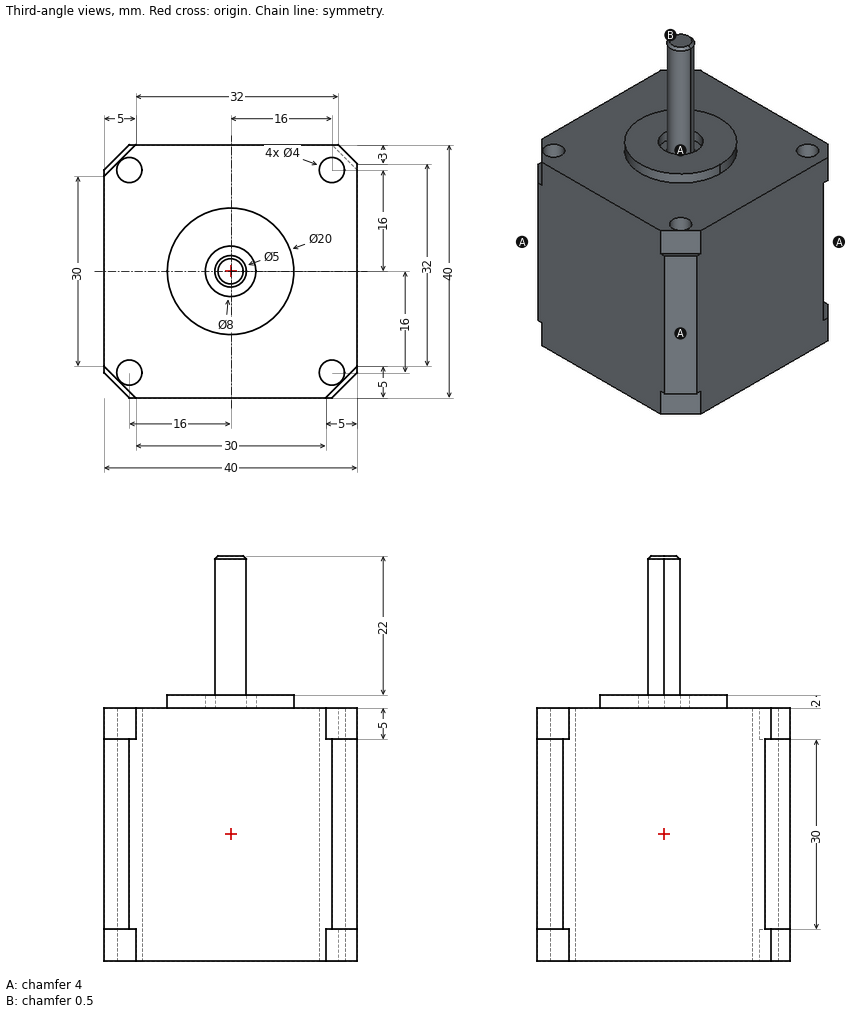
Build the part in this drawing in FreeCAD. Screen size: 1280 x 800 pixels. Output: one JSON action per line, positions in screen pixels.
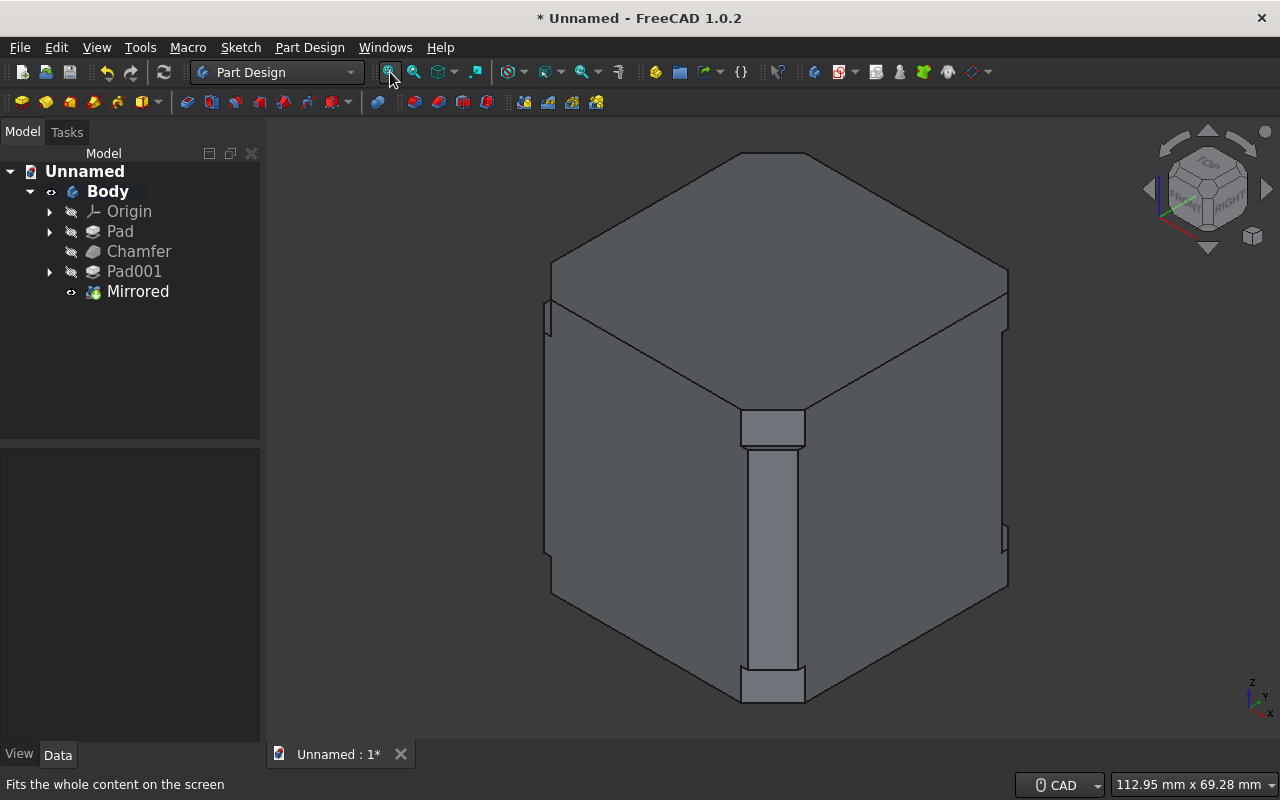
{"action": "left_click", "coordinate": [773, 280]}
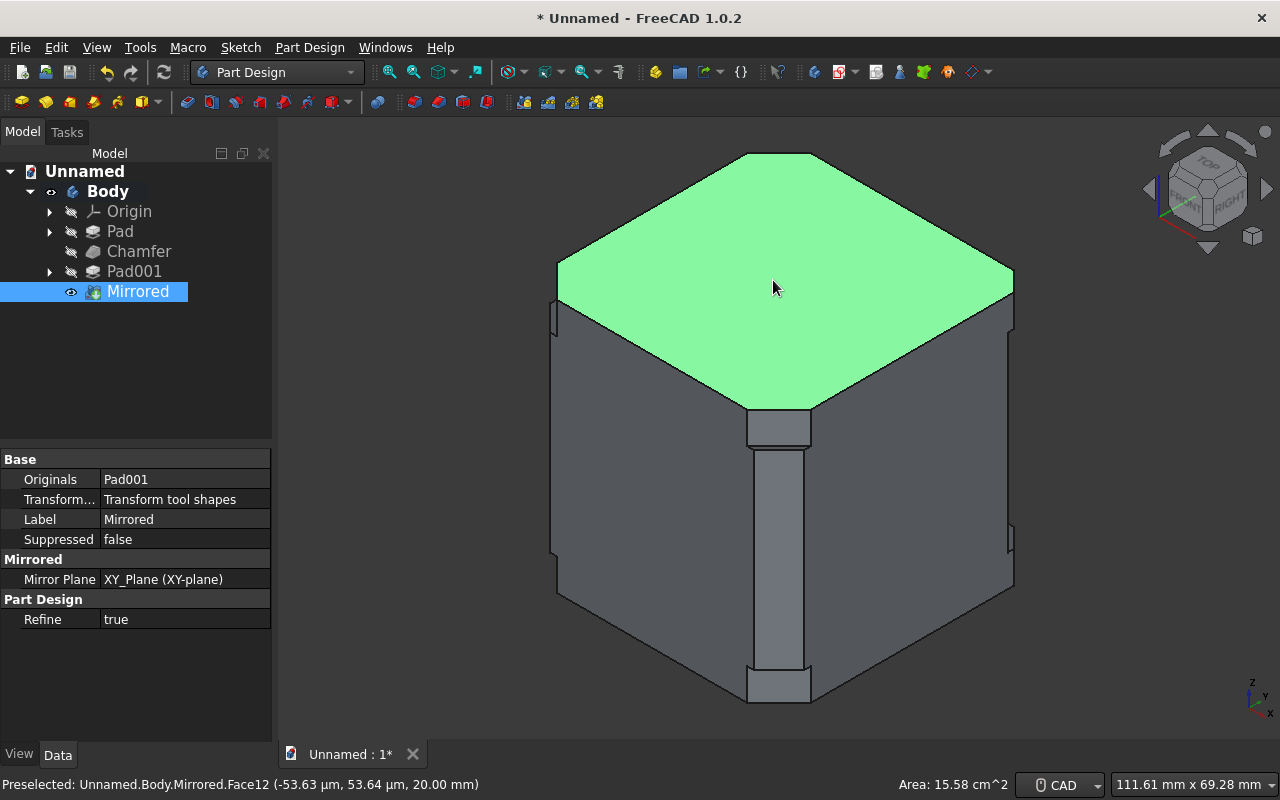
{"action": "left_click", "coordinate": [840, 72]}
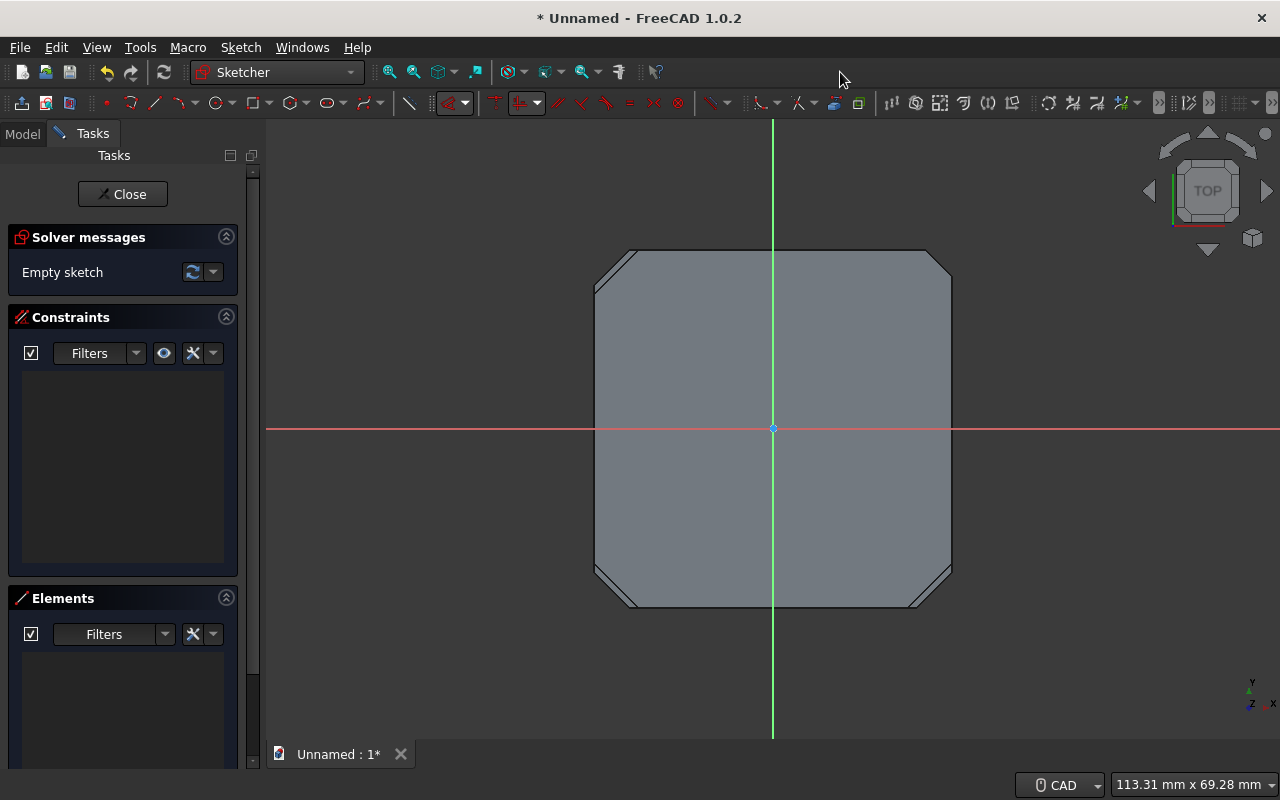
{"action": "scroll", "coordinate": [829, 429], "scroll_direction": "up", "scroll_amount": 4}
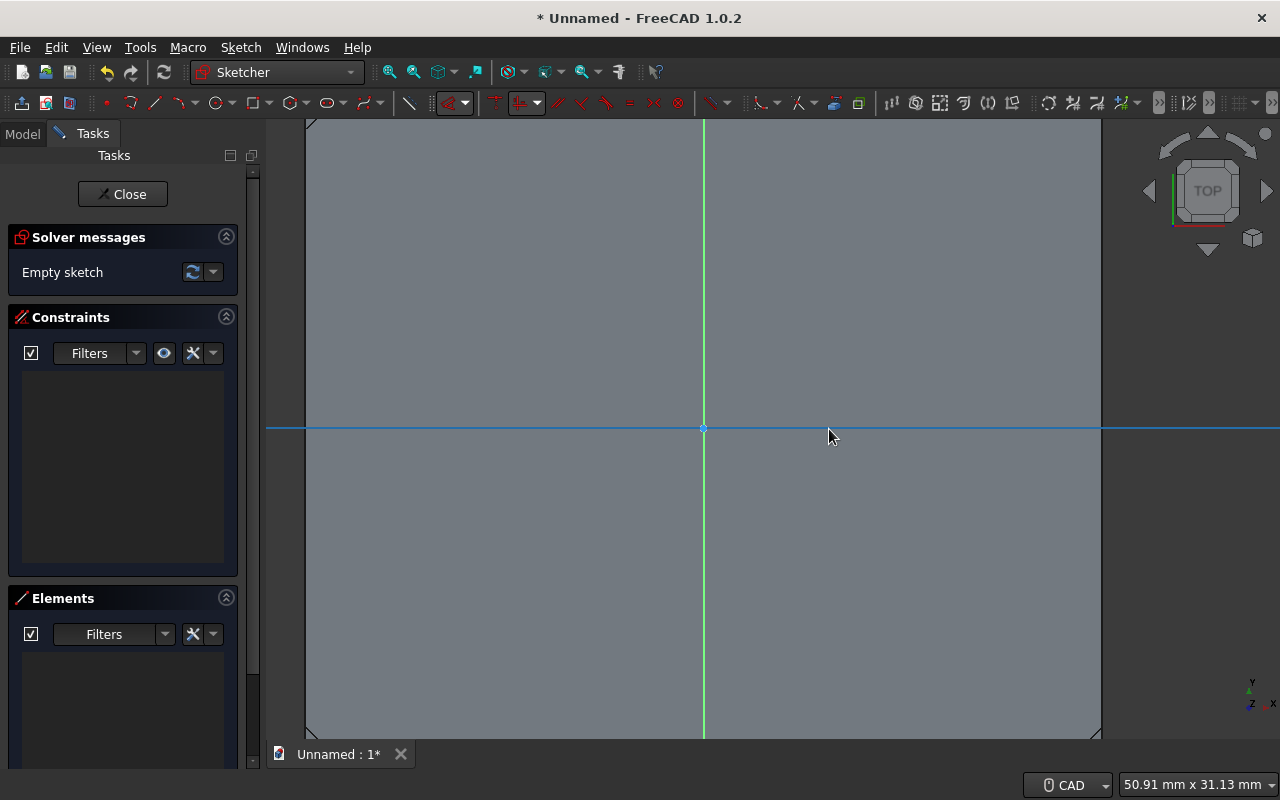
{"action": "left_click", "coordinate": [216, 104]}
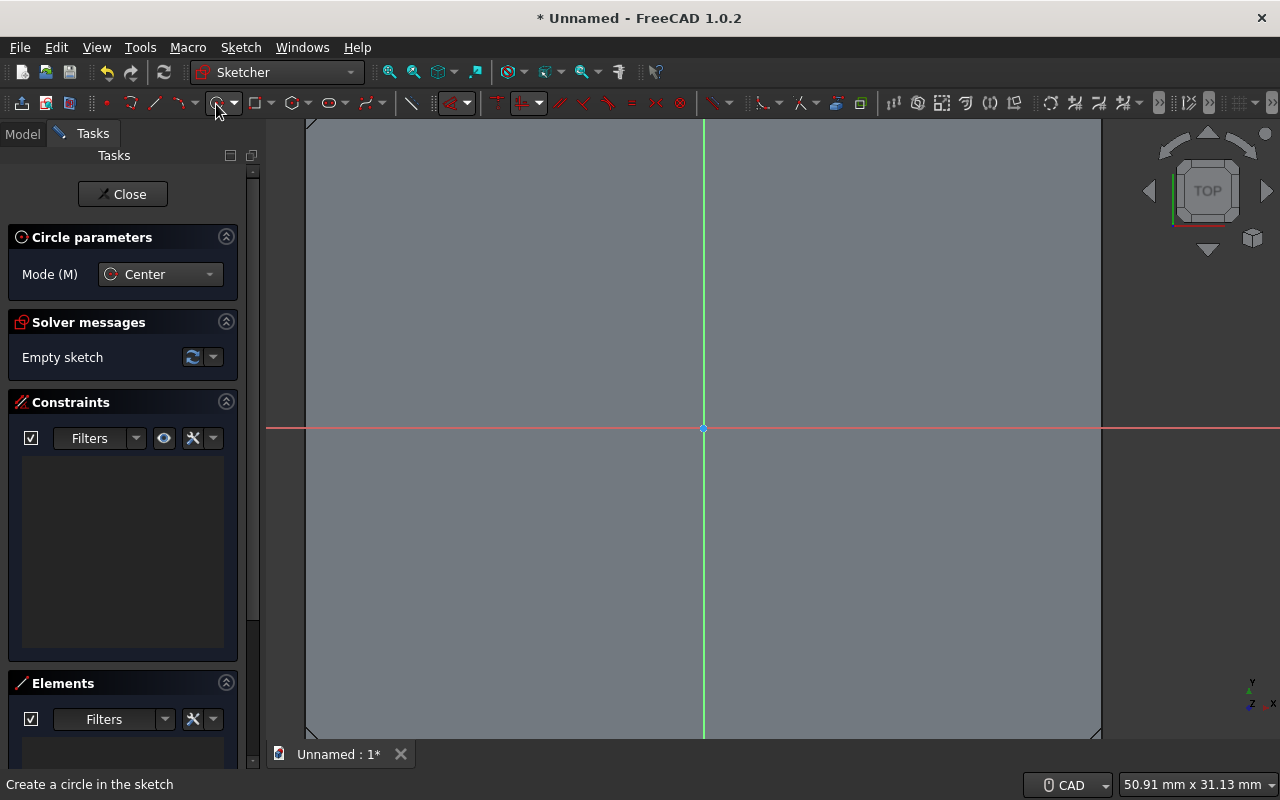
{"action": "left_click", "coordinate": [704, 428]}
{"action": "mouse_move", "coordinate": [845, 288]}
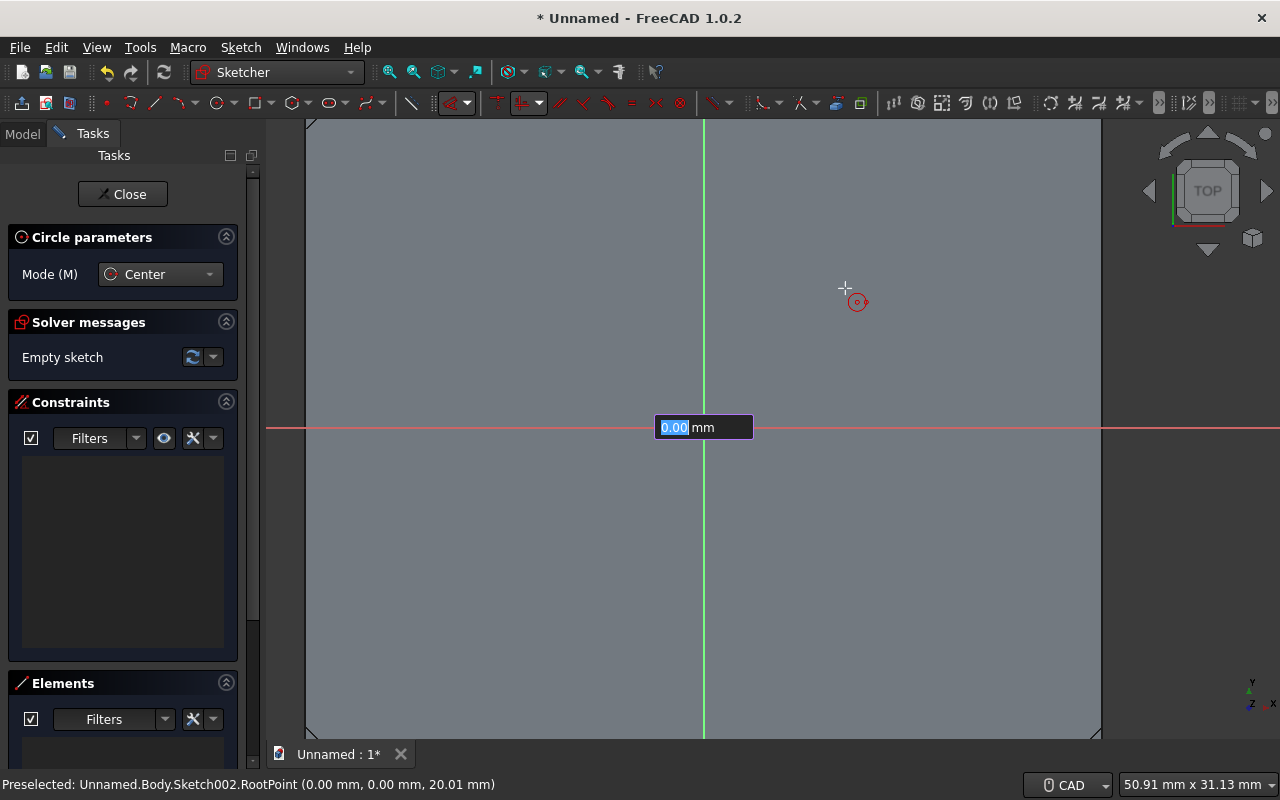
{"action": "type", "text": "20"}
{"action": "key", "text": "Return"}
{"action": "key", "text": "Escape"}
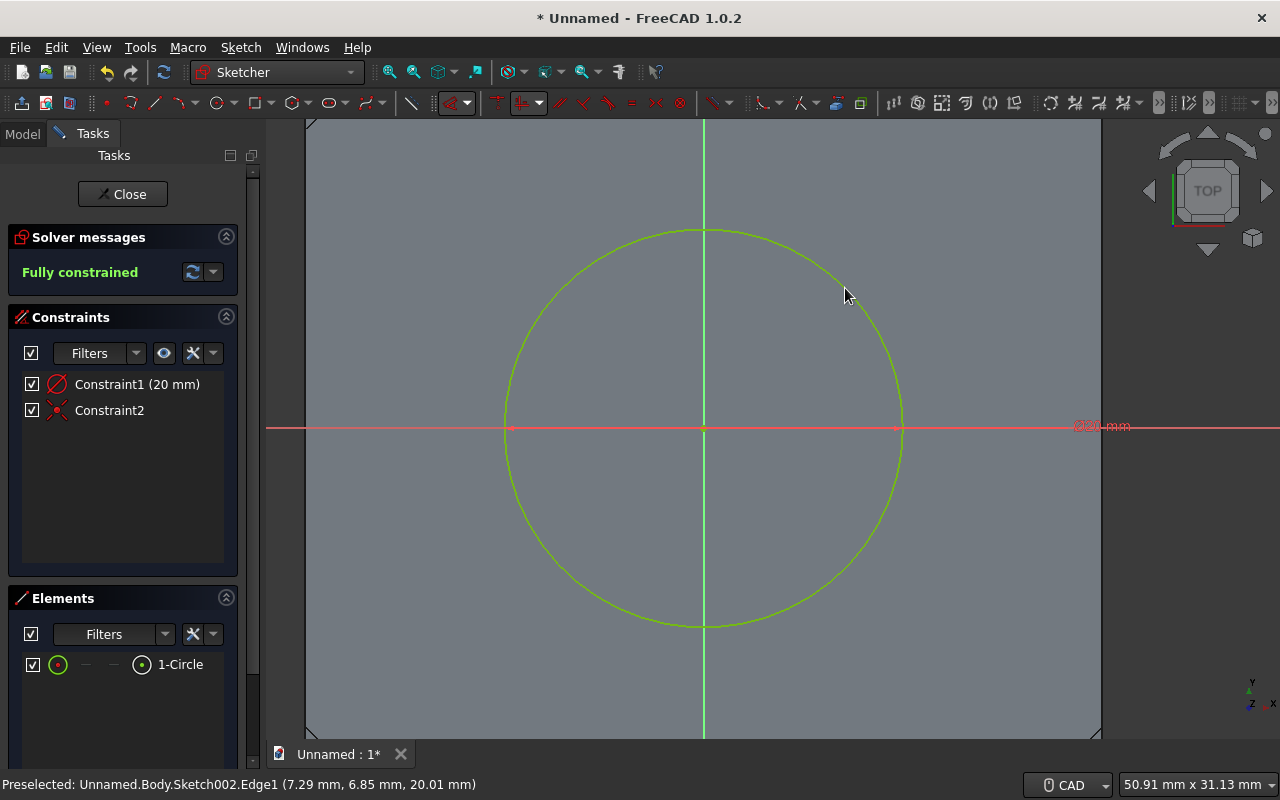
{"action": "left_click", "coordinate": [123, 194]}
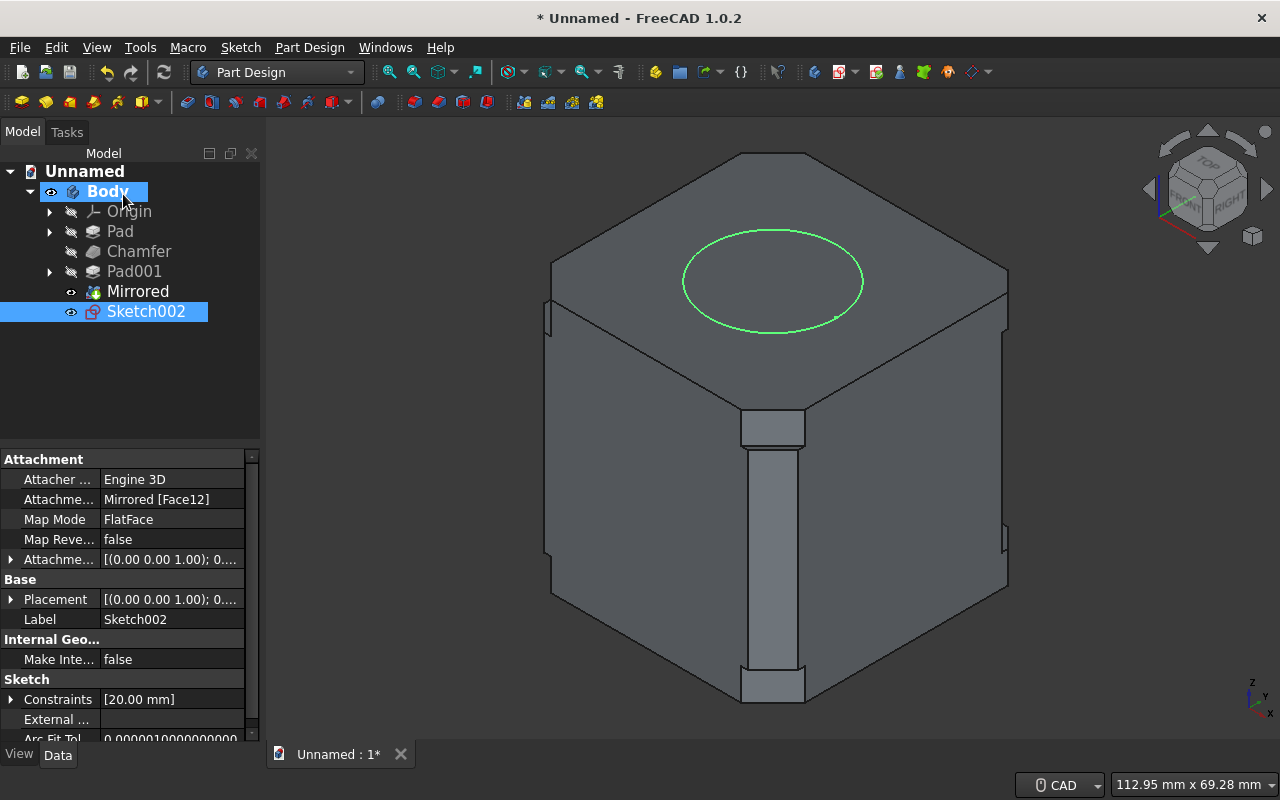
{"action": "left_click", "coordinate": [22, 102]}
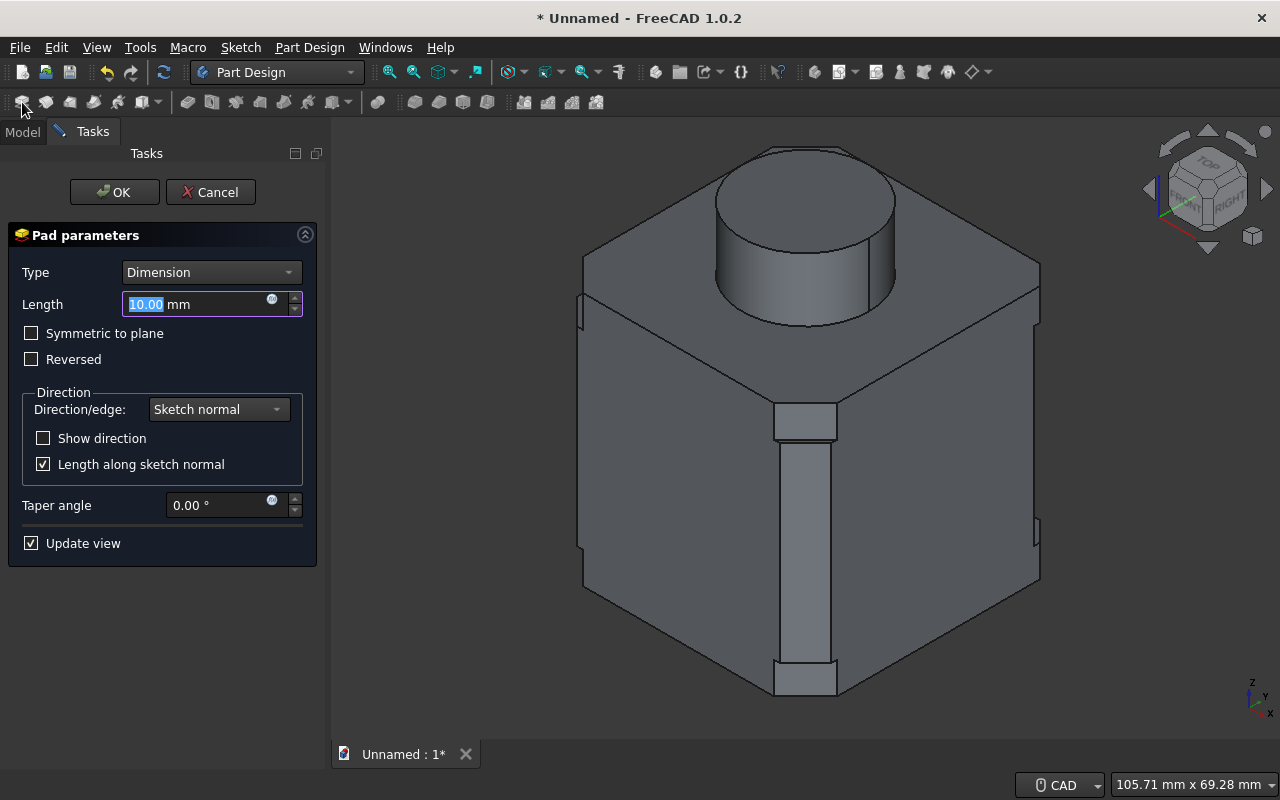
{"action": "type", "text": "2"}
{"action": "key", "text": "Tab"}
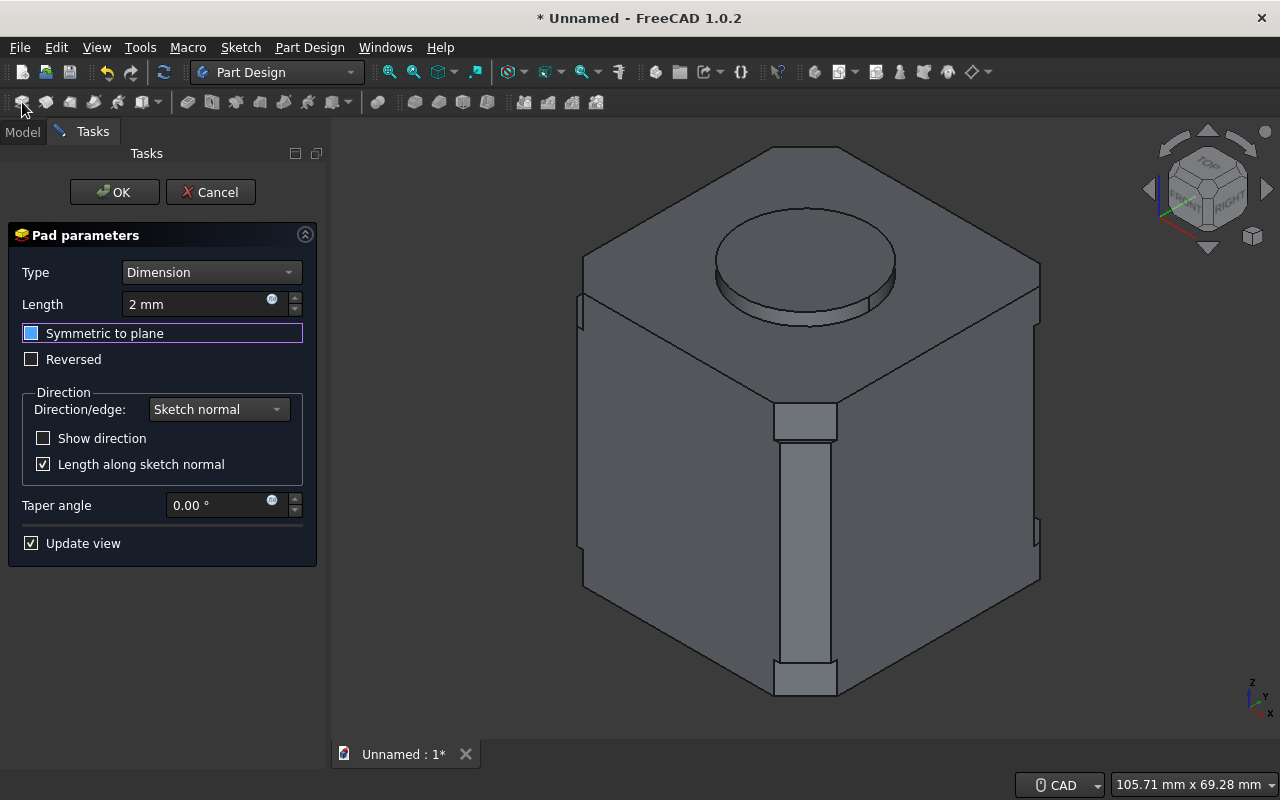
{"action": "left_click", "coordinate": [115, 192]}